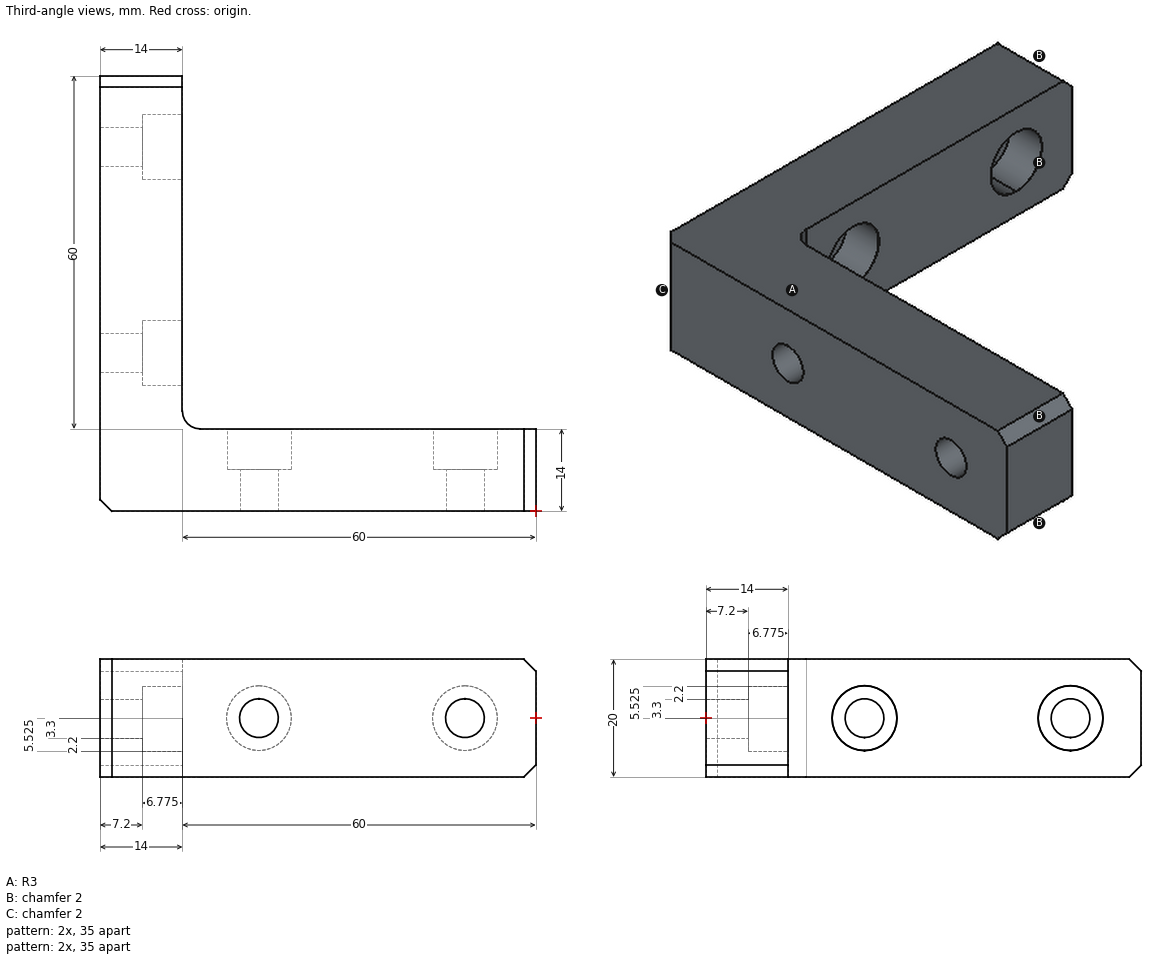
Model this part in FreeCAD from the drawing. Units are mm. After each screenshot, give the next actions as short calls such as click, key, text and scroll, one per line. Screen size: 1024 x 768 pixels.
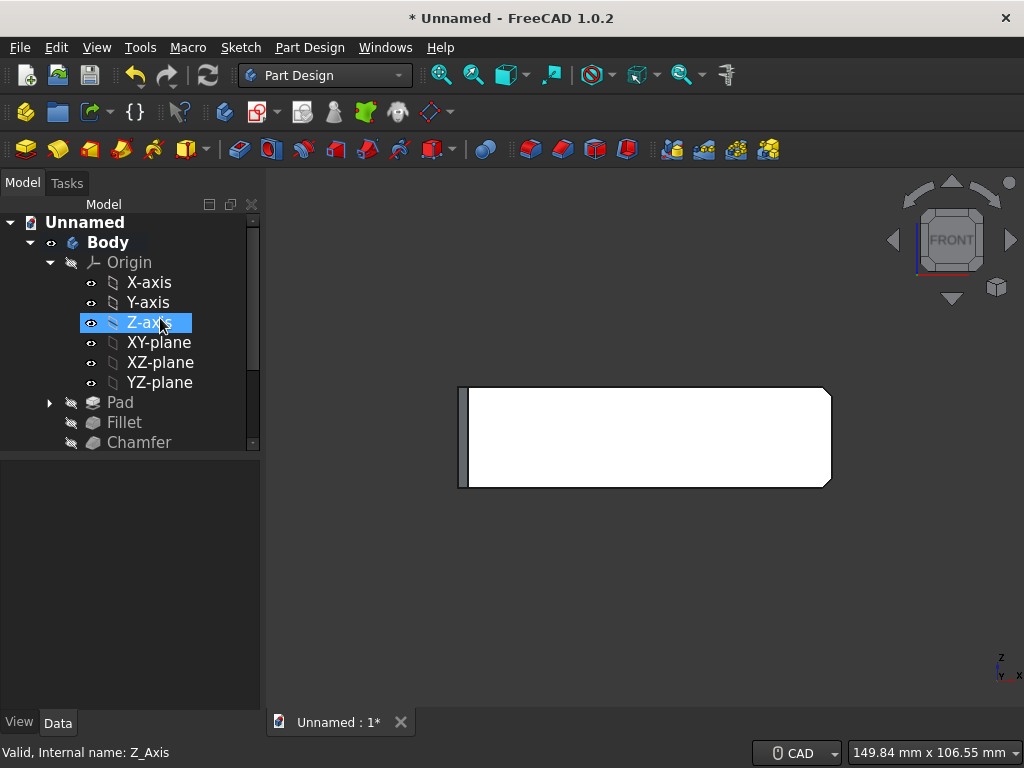
click(136, 383)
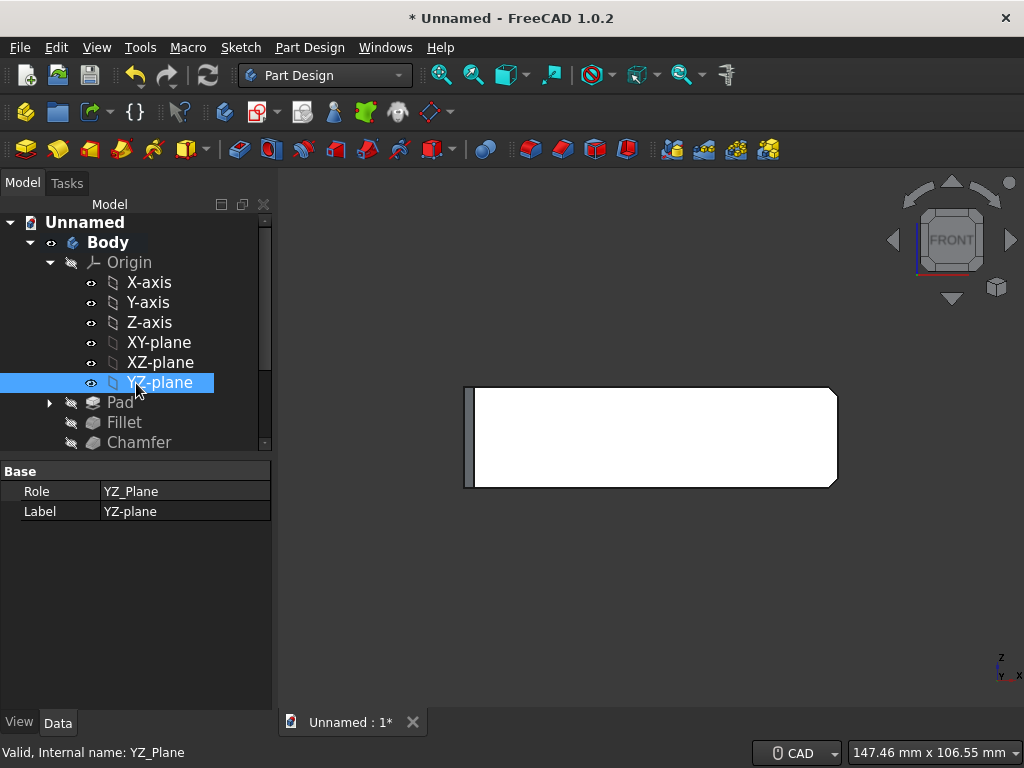
click(430, 112)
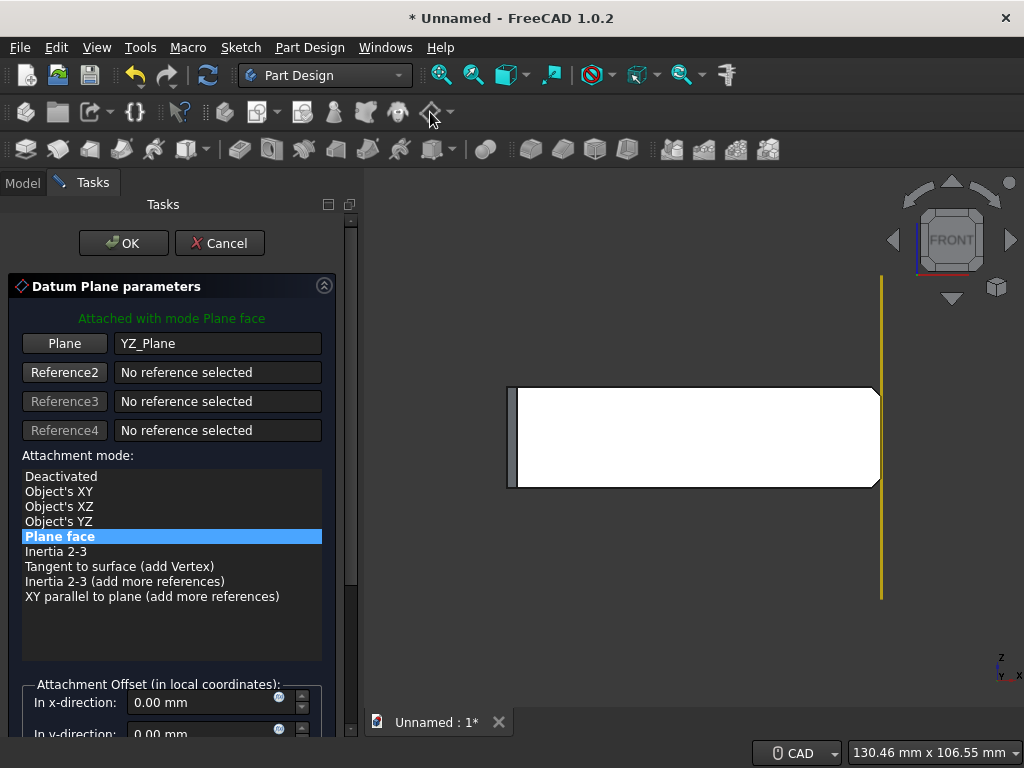
scroll(351, 475, down, 2)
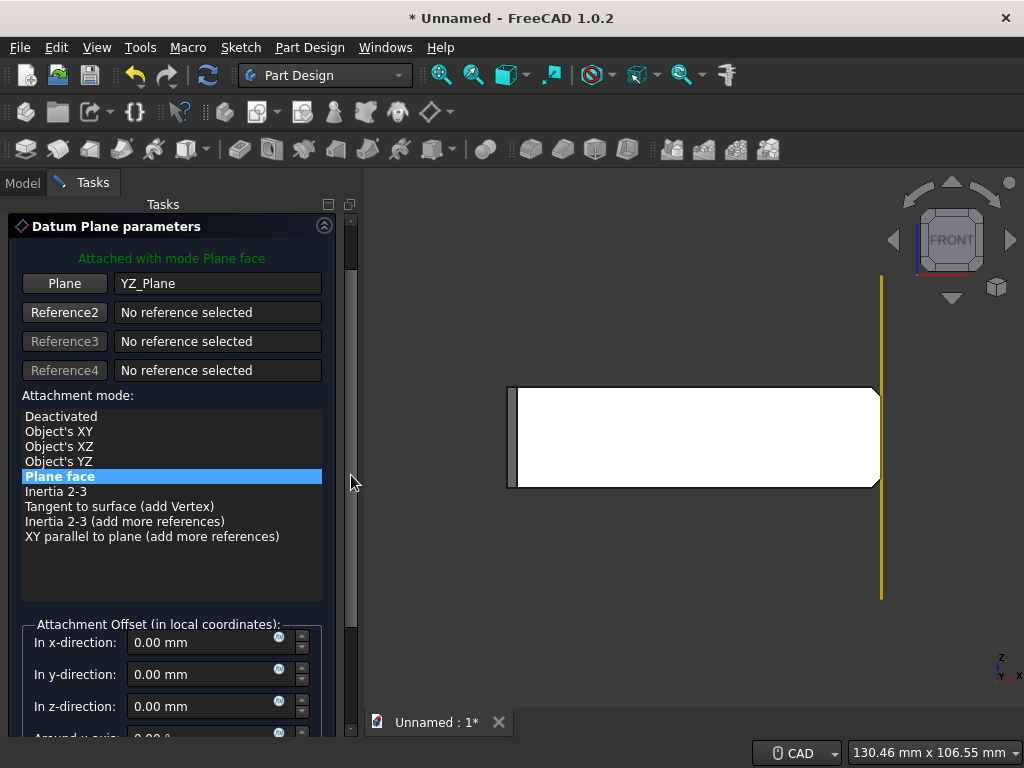
triple_click(210, 646)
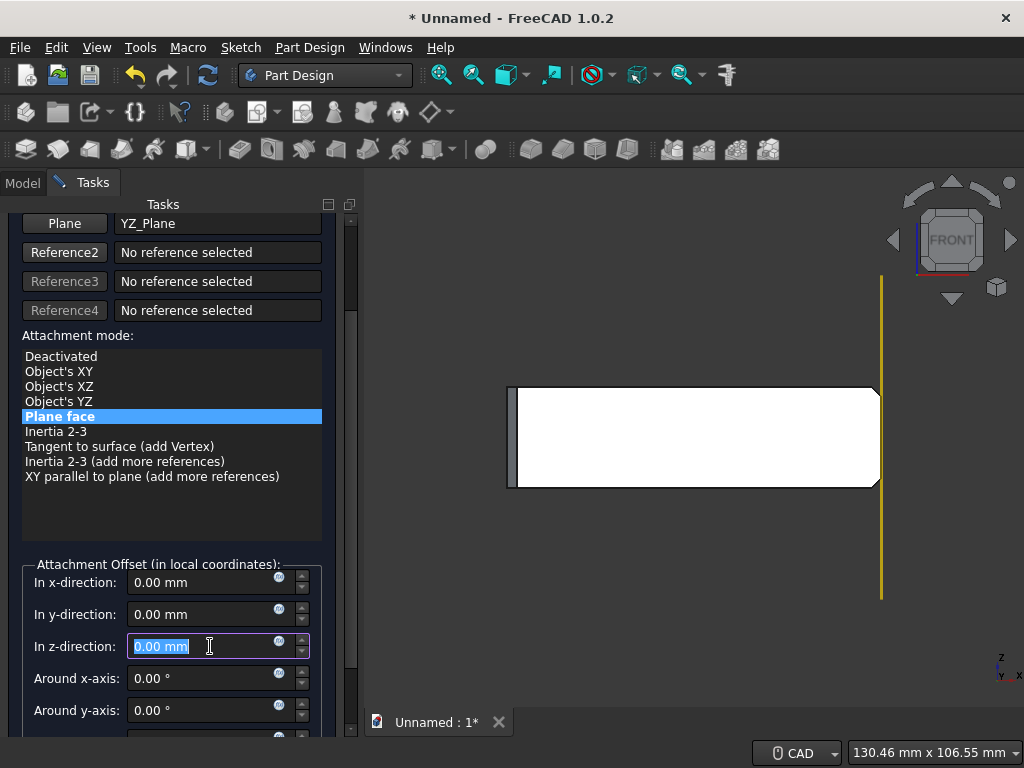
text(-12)
key(Tab)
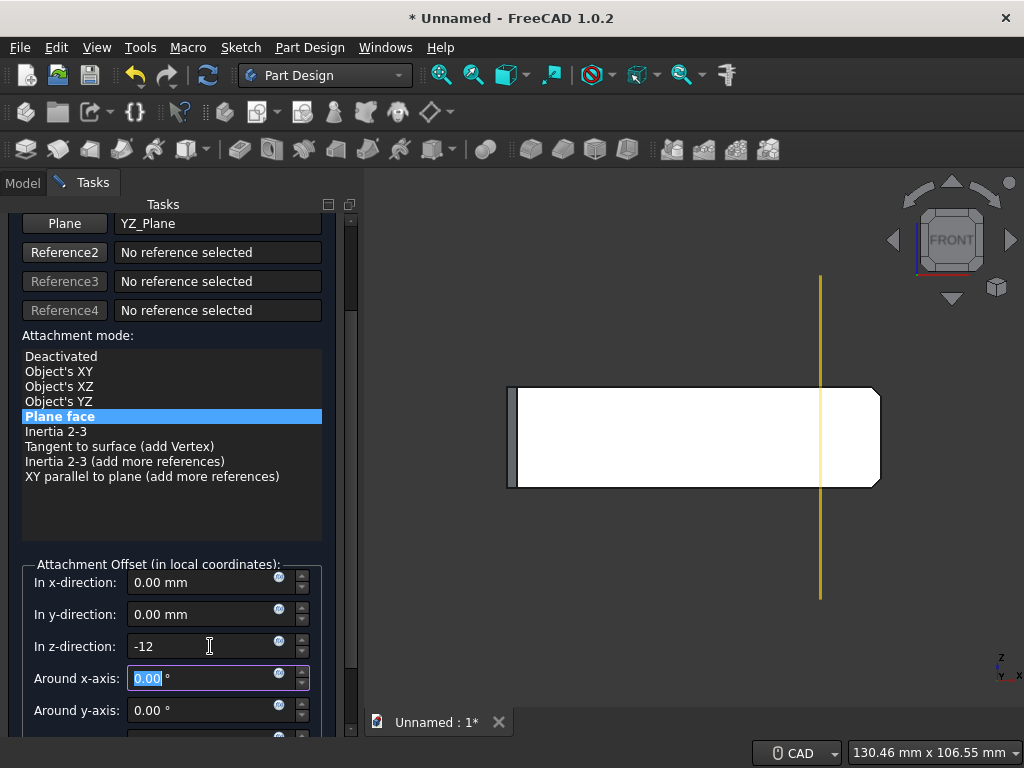
scroll(351, 475, up, 3)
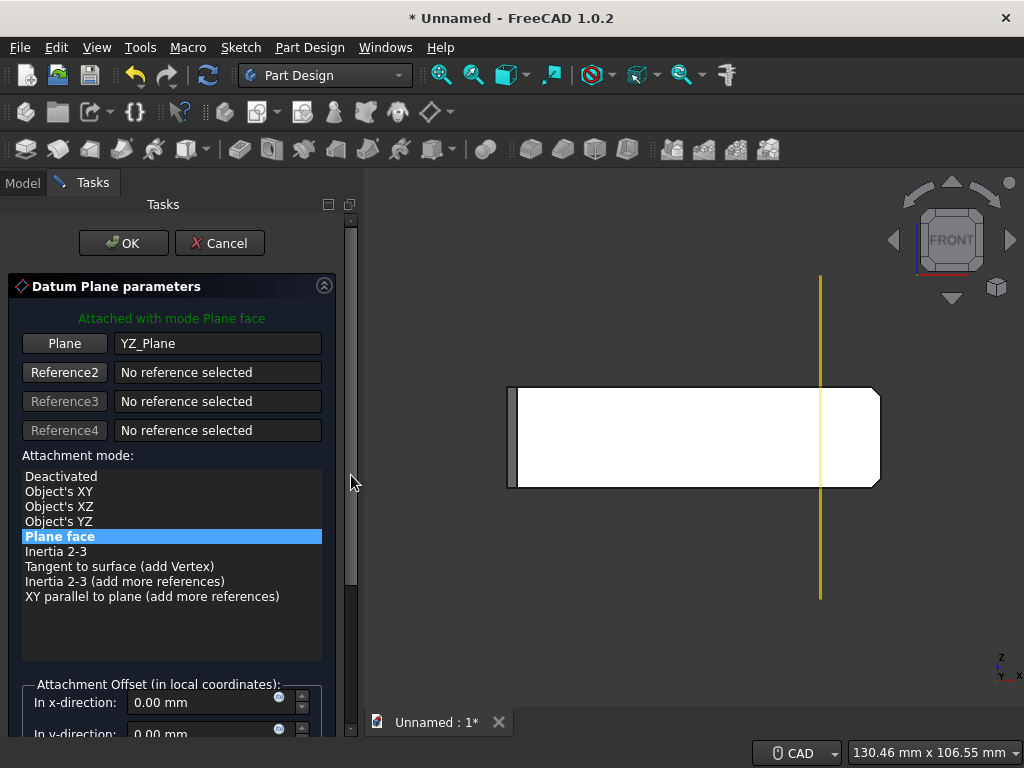
click(124, 243)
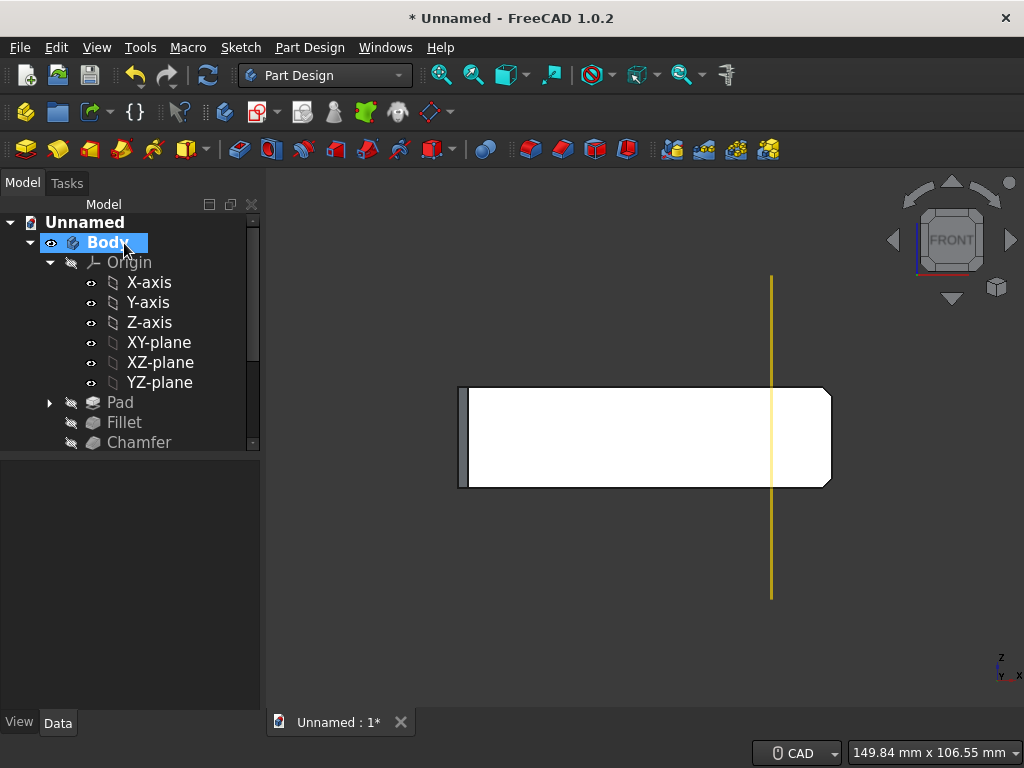
scroll(100, 338, down, 3)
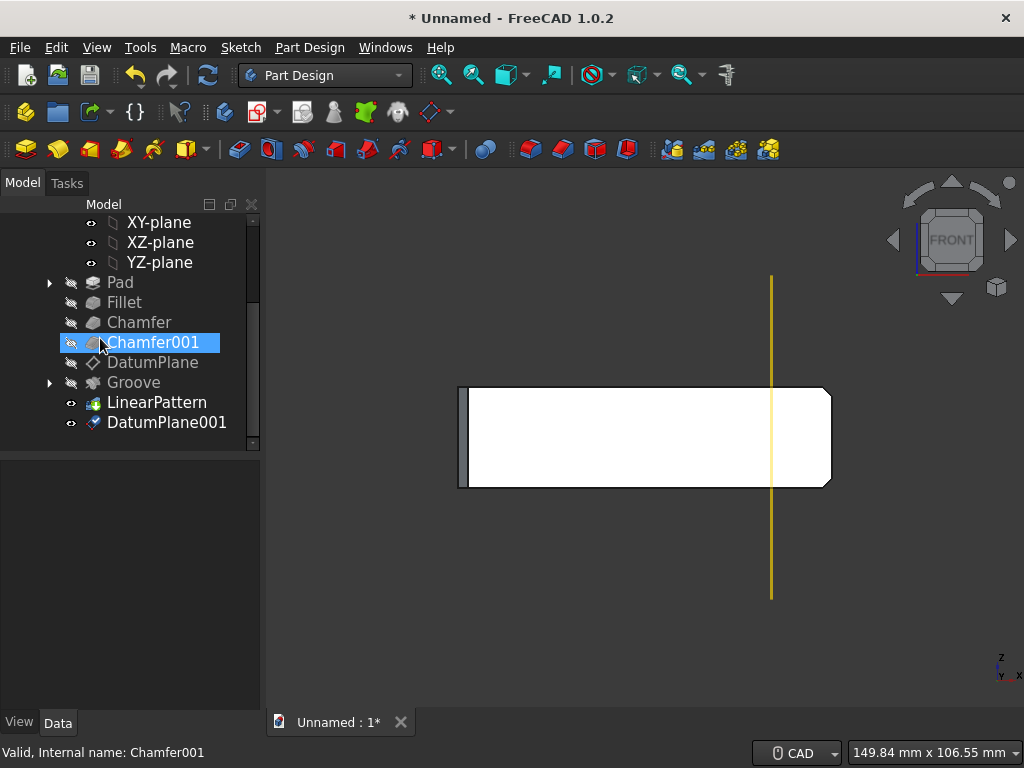
click(116, 423)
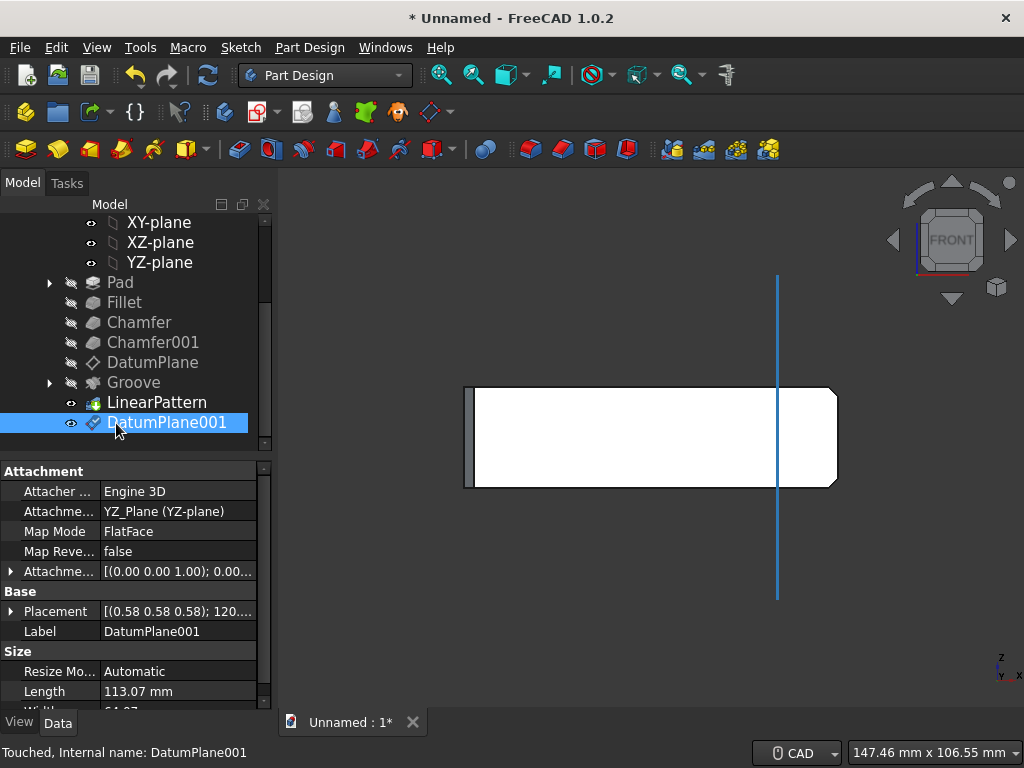
click(258, 112)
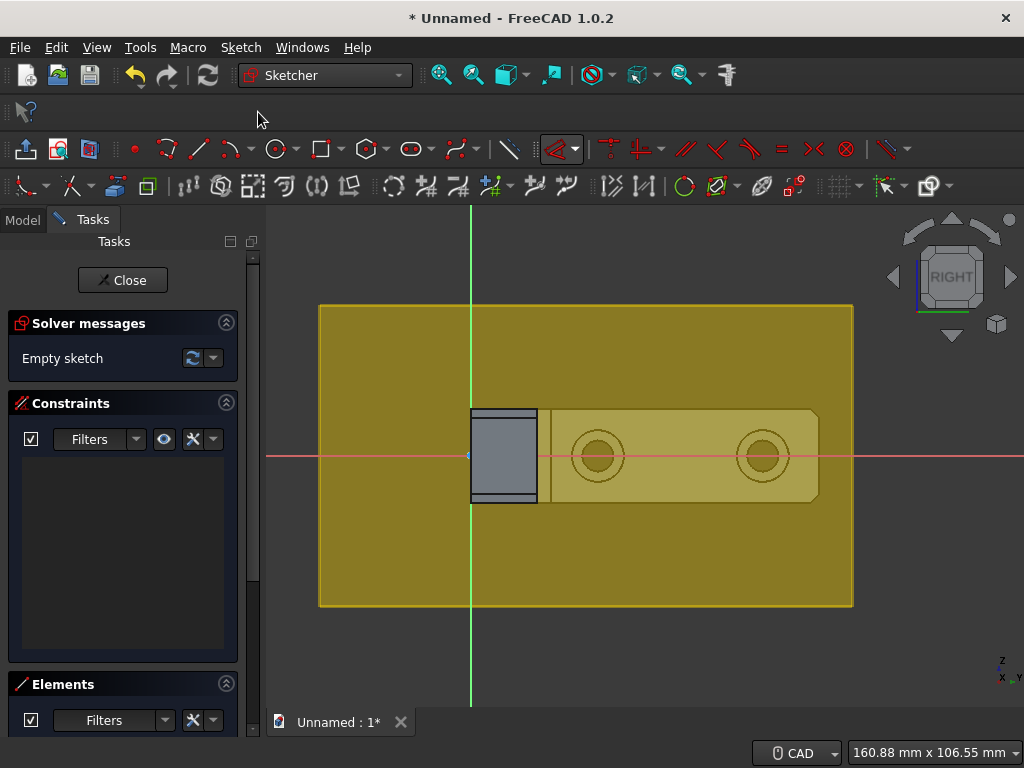
click(90, 150)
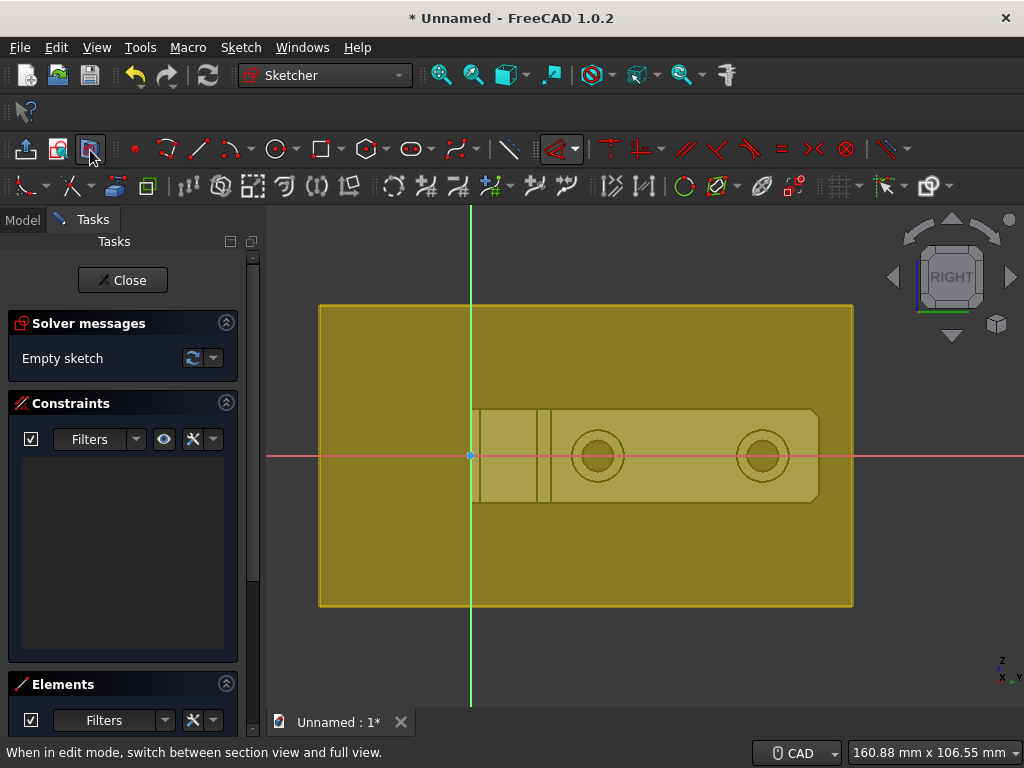
scroll(489, 440, up, 9)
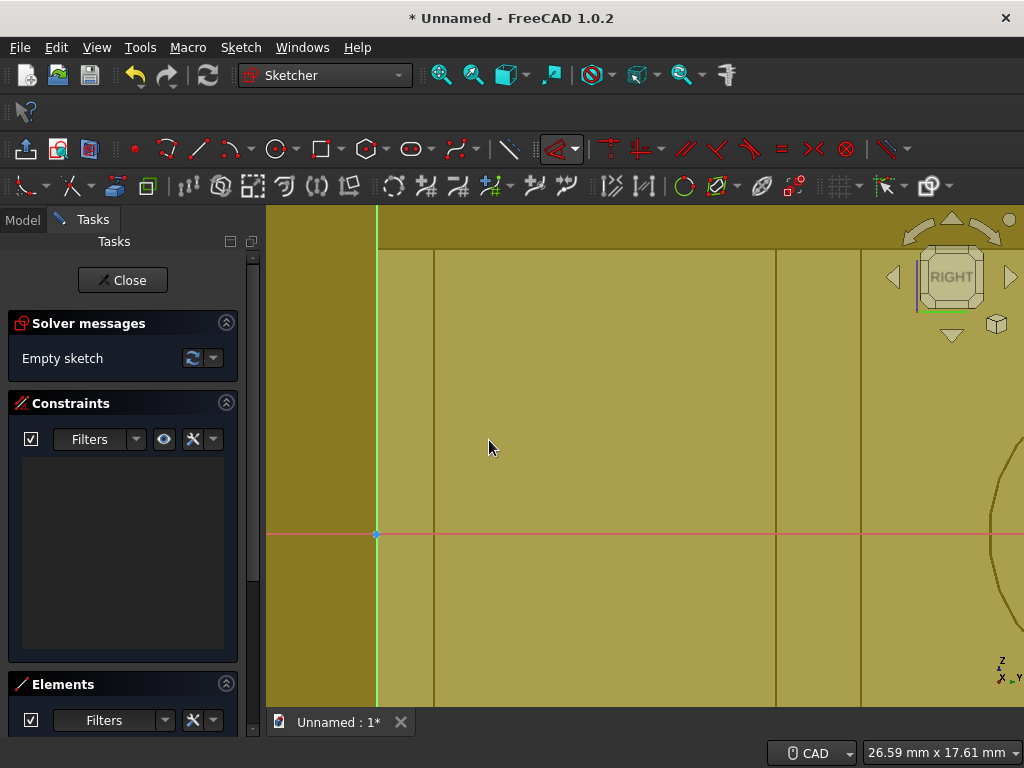
click(168, 150)